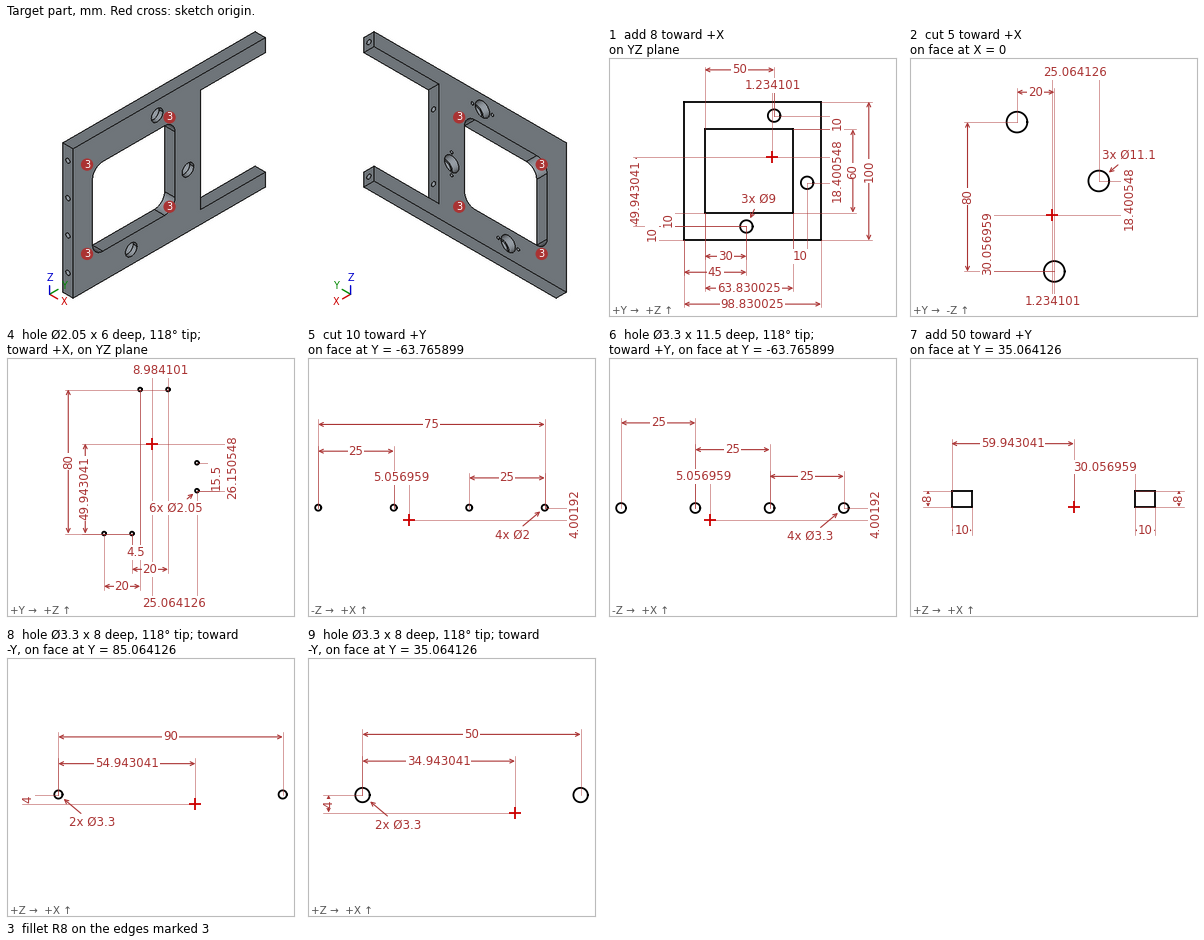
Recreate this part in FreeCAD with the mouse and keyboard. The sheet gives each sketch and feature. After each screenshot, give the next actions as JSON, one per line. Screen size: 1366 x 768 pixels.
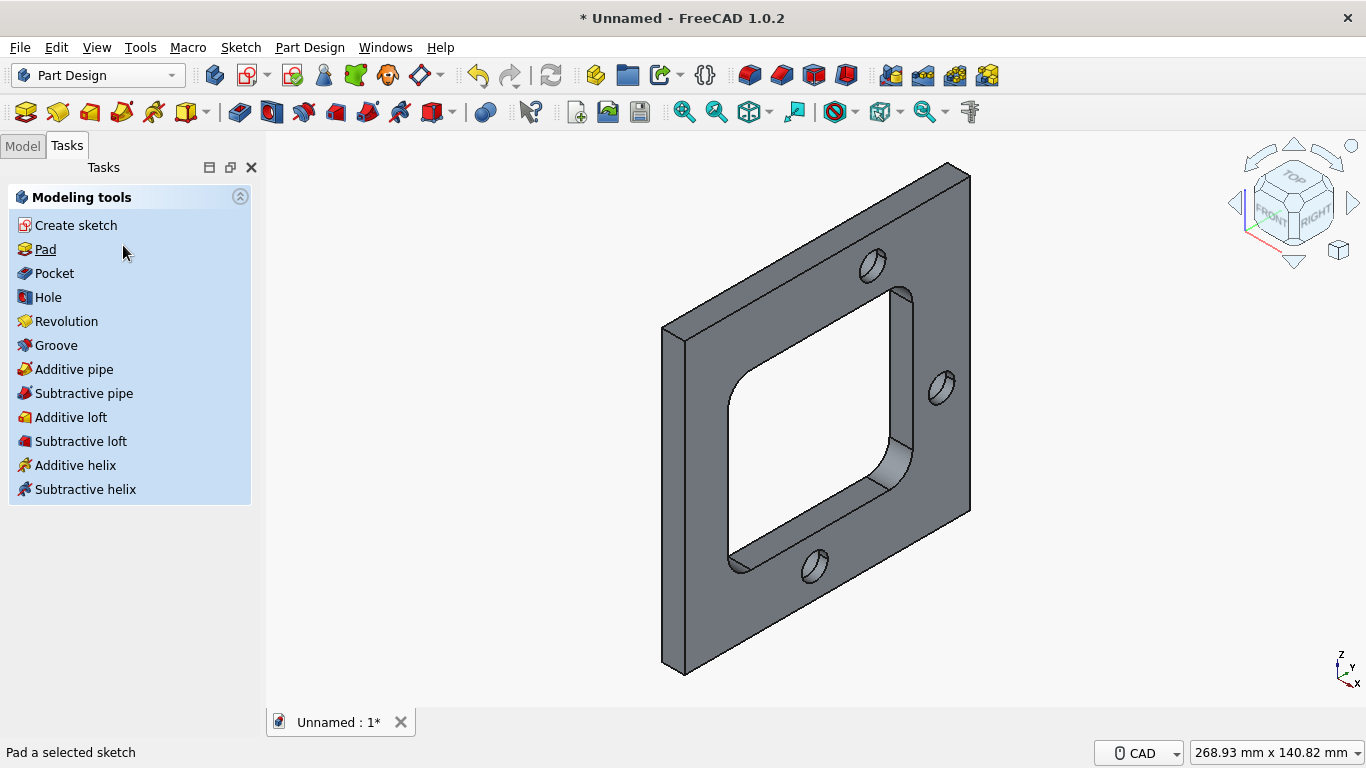
{"action": "left_click", "coordinate": [272, 112]}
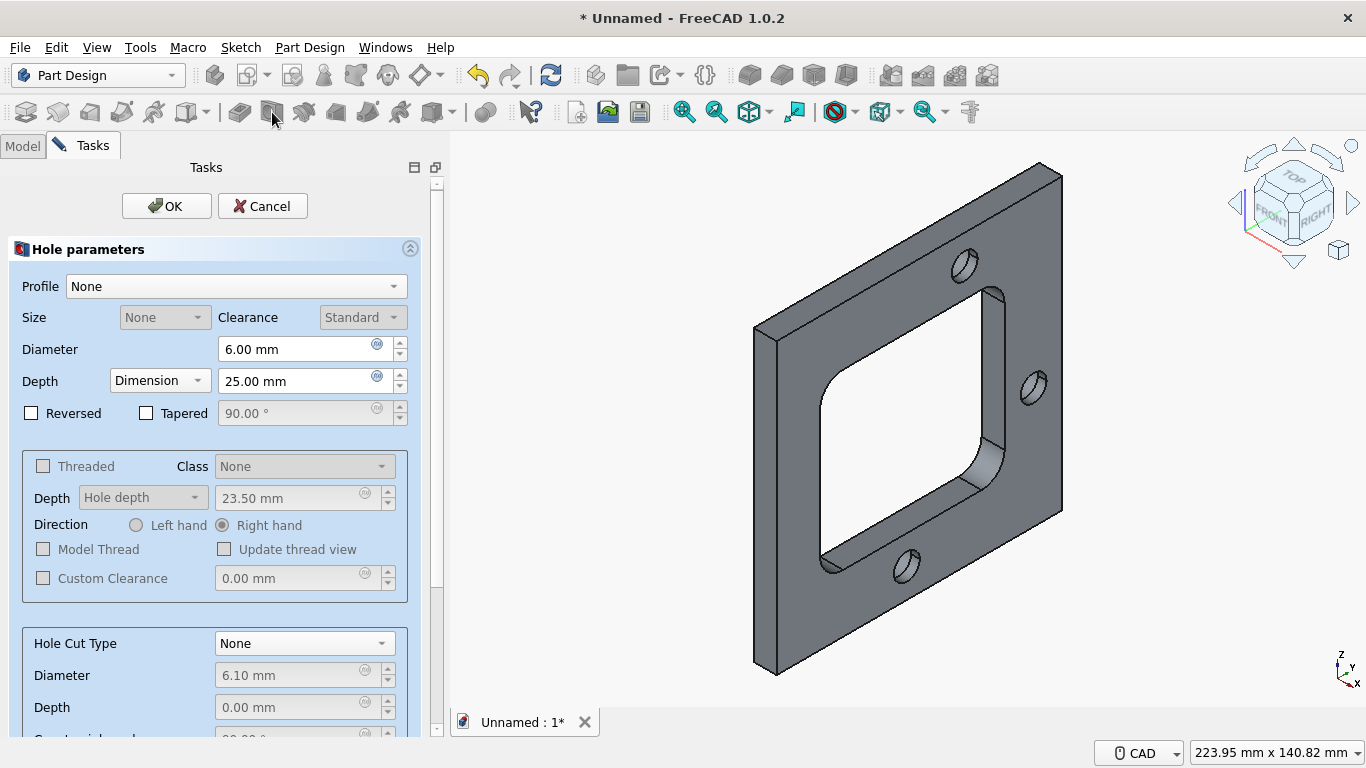
{"action": "triple_click", "coordinate": [305, 349]}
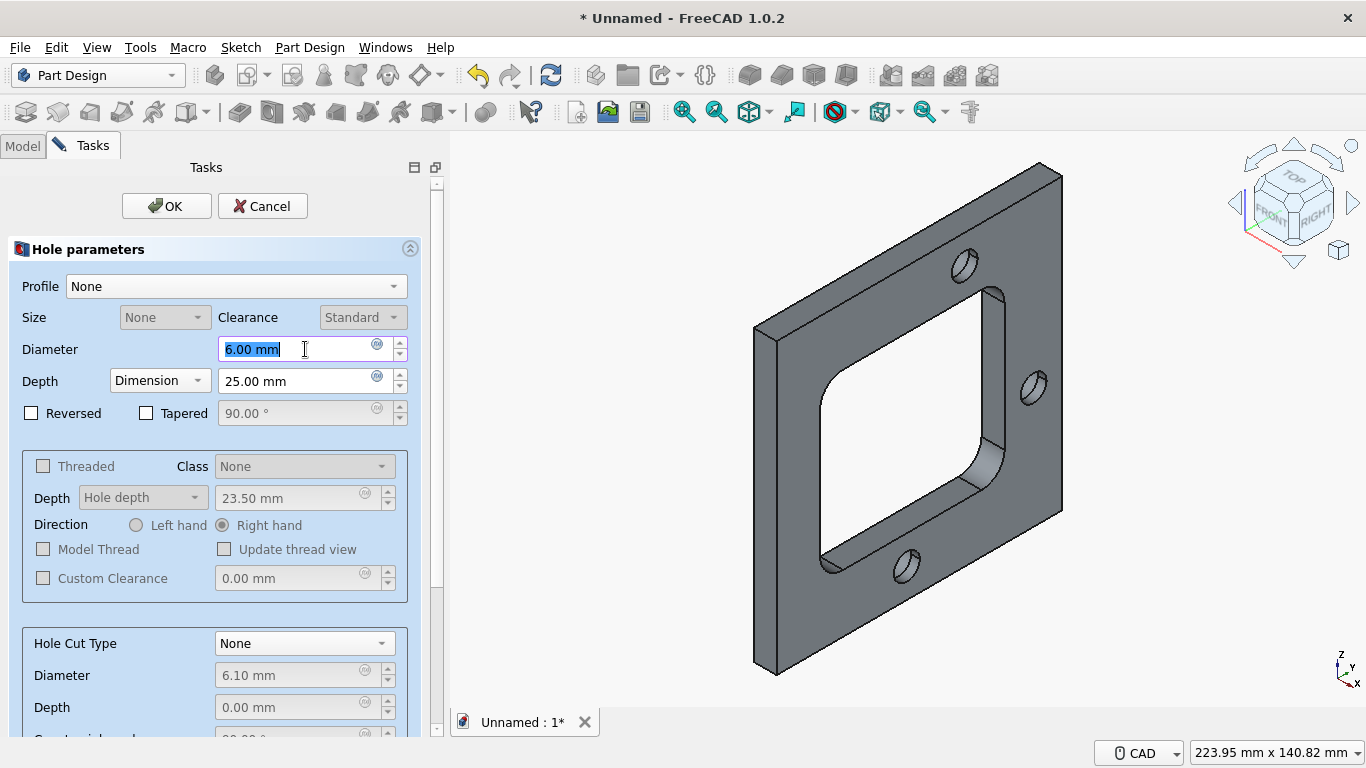
{"action": "type", "text": "2.05"}
{"action": "key", "text": "Tab"}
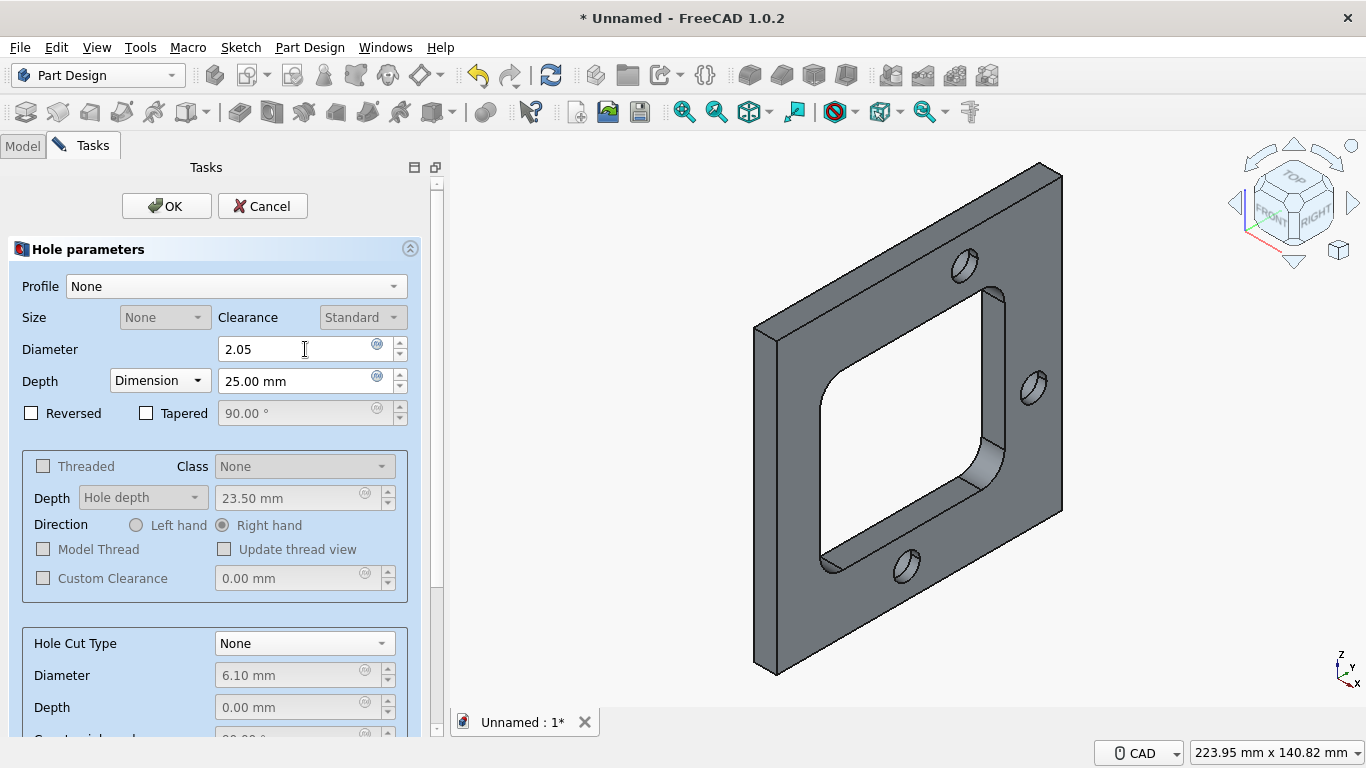
{"action": "triple_click", "coordinate": [305, 381]}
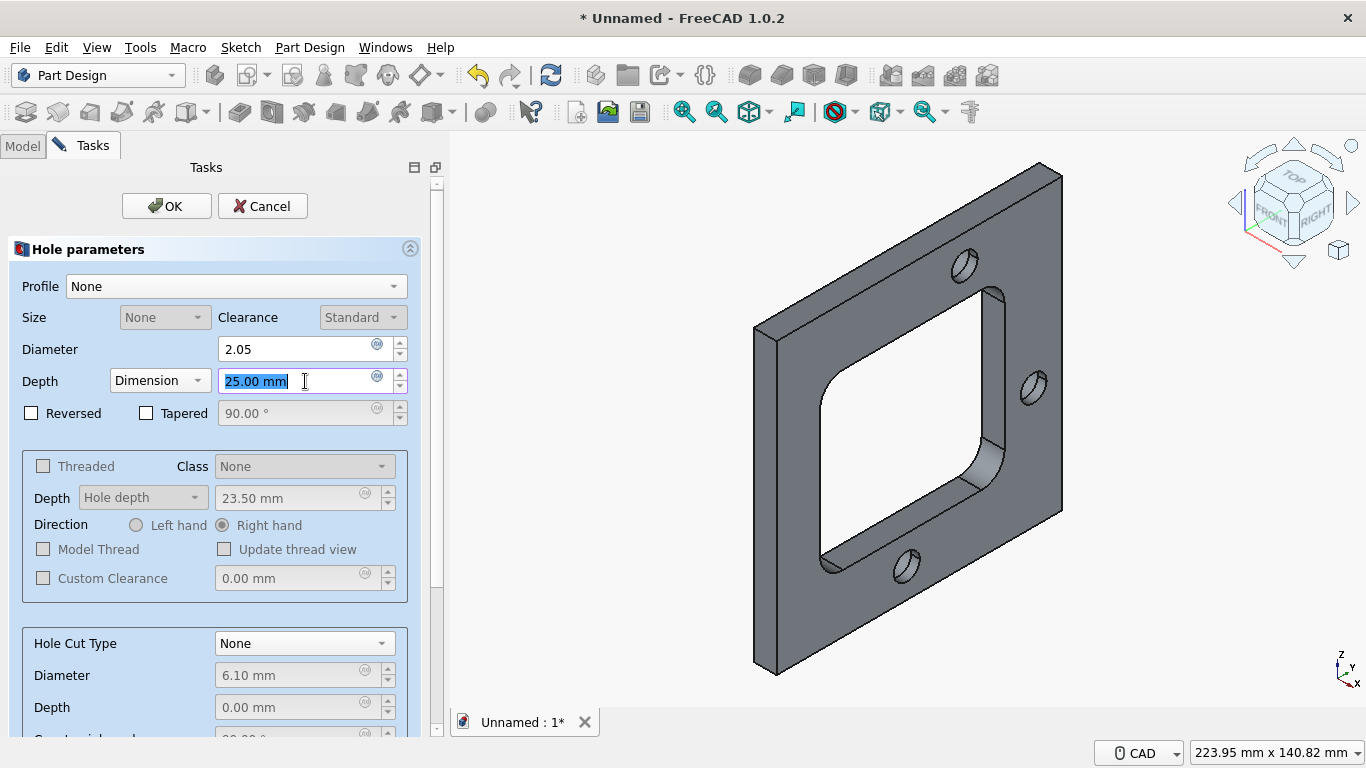
{"action": "type", "text": "6"}
{"action": "key", "text": "Tab"}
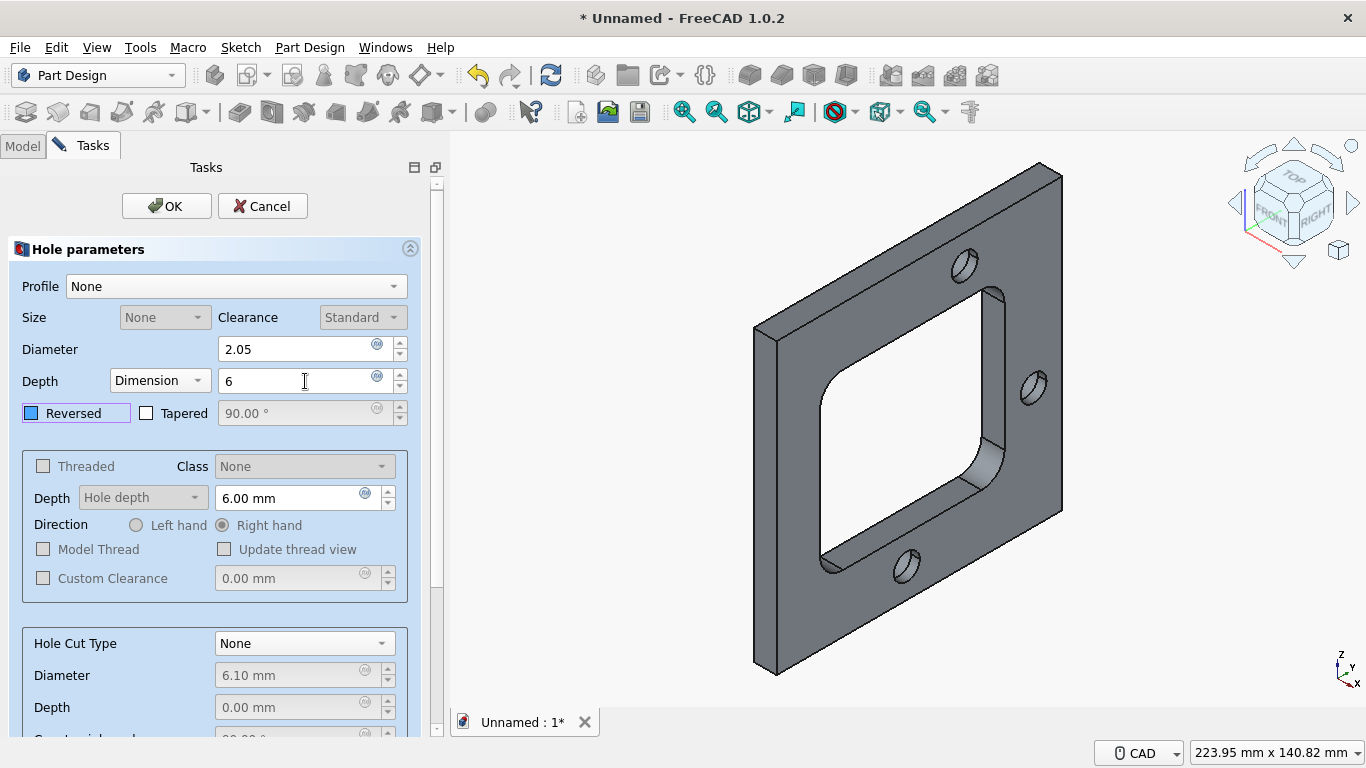
{"action": "left_click", "coordinate": [30, 413]}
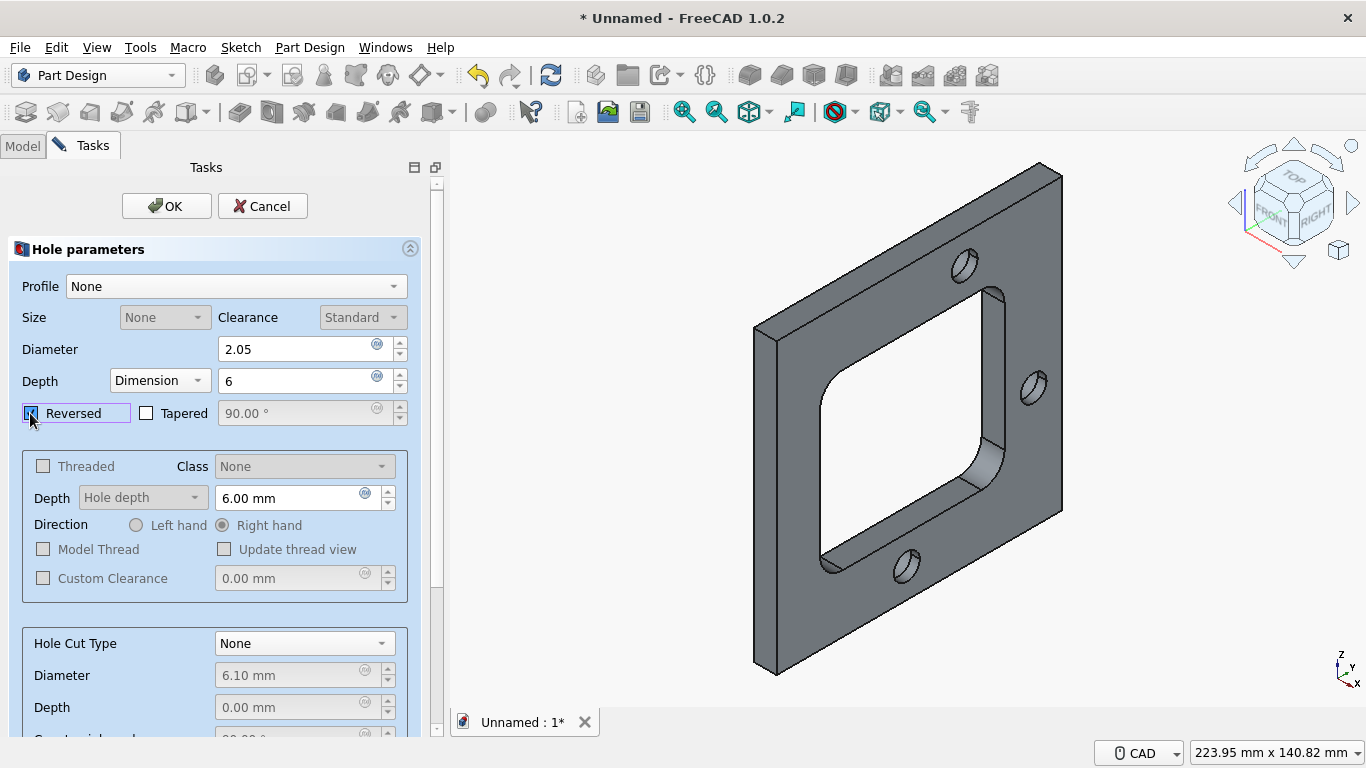
{"action": "left_click", "coordinate": [167, 206]}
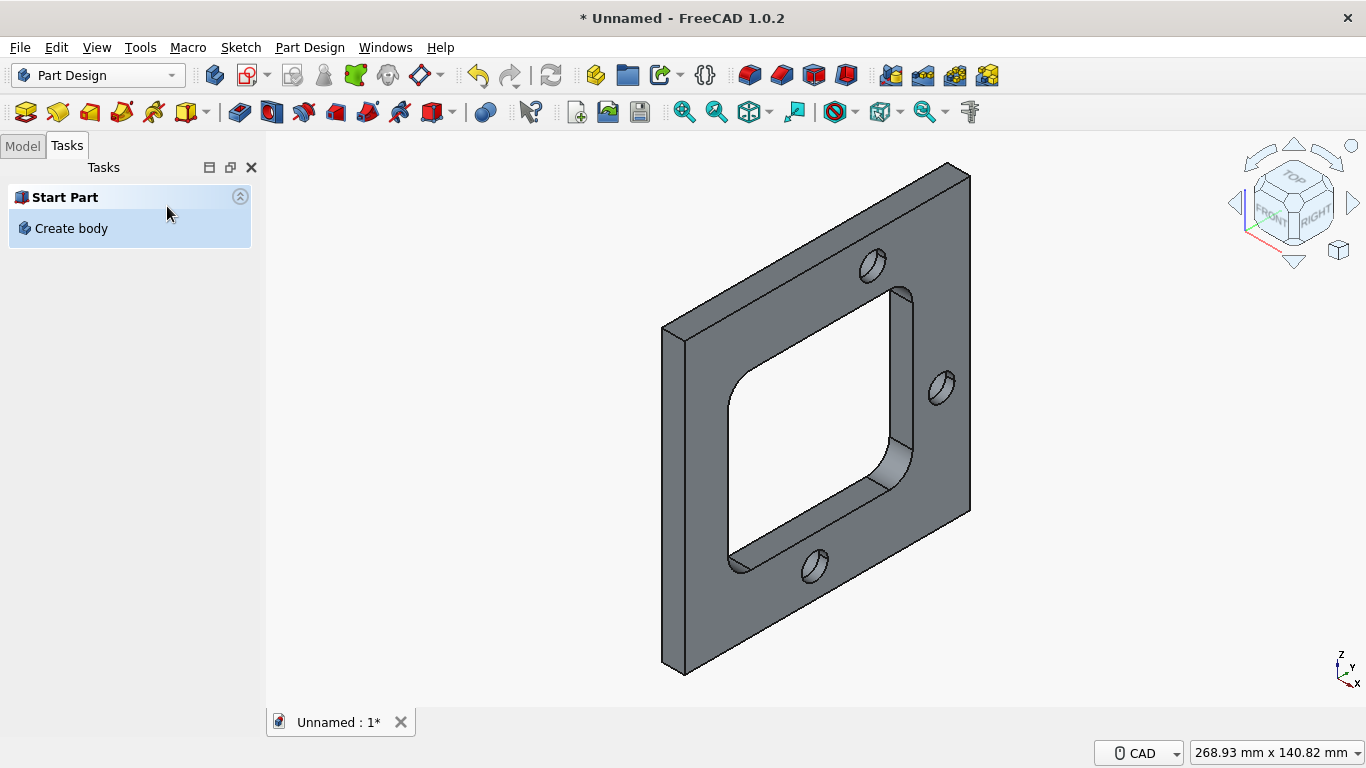
{"action": "left_click", "coordinate": [673, 644]}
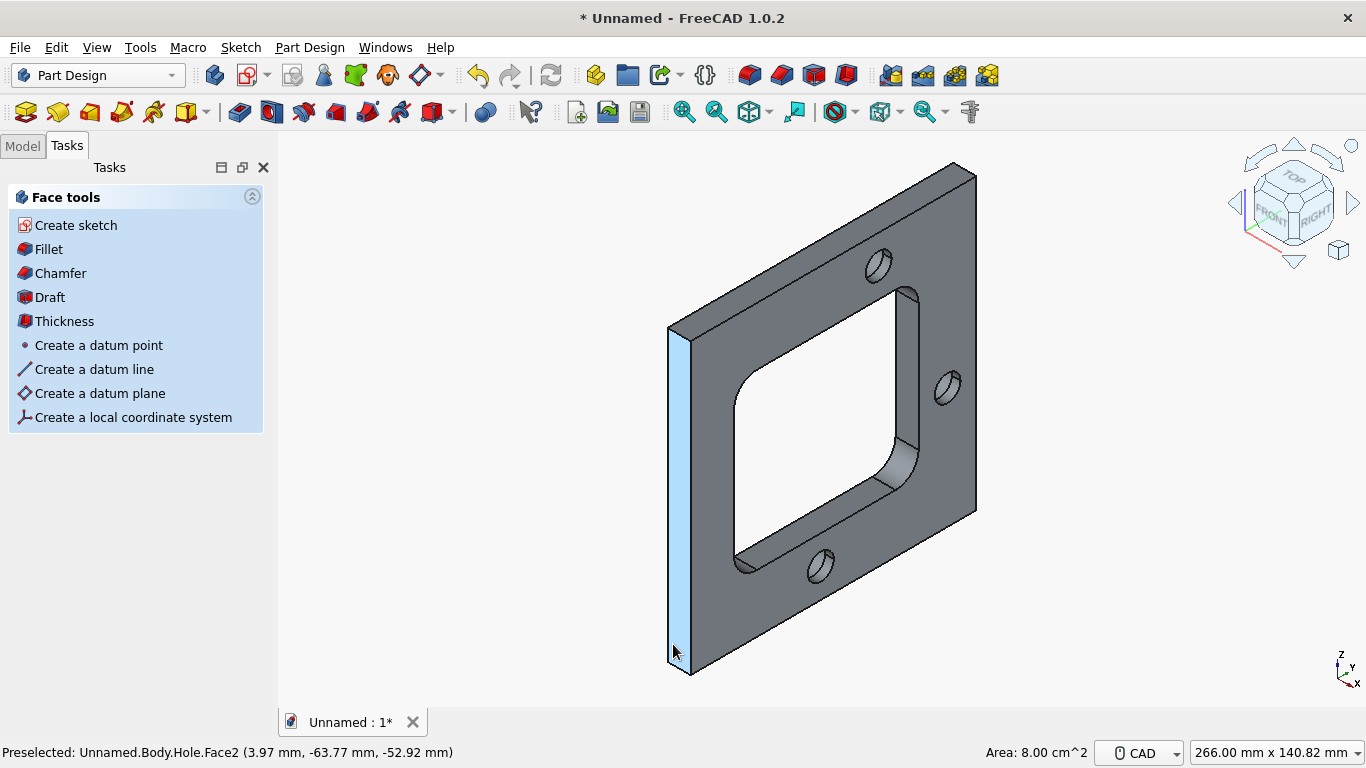
{"action": "left_click", "coordinate": [248, 76]}